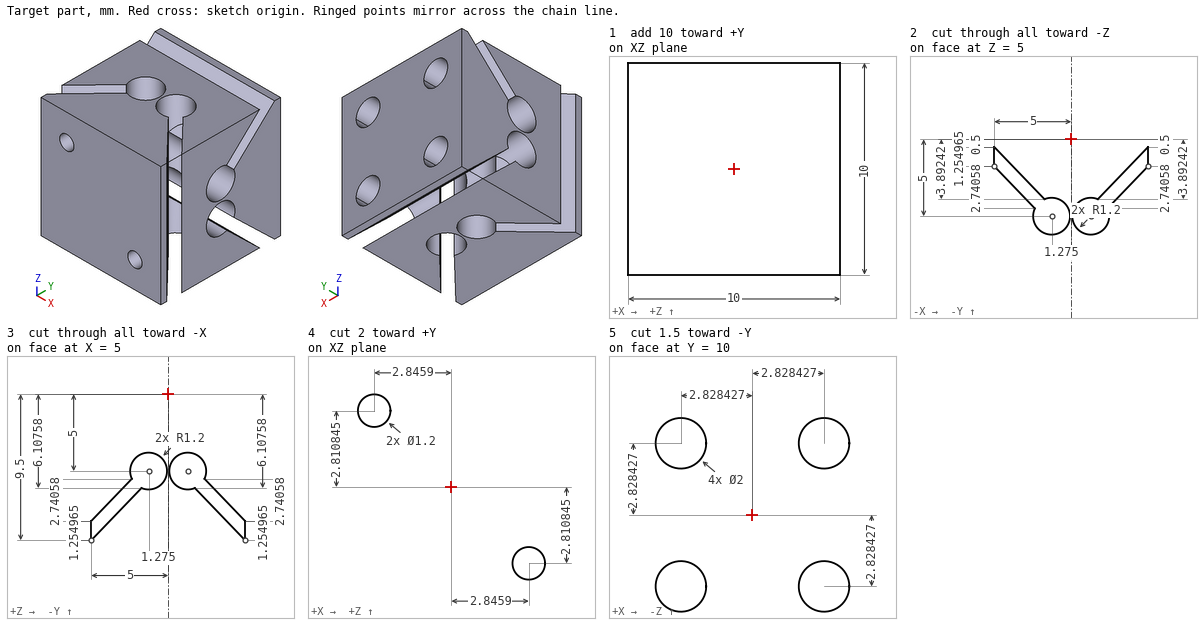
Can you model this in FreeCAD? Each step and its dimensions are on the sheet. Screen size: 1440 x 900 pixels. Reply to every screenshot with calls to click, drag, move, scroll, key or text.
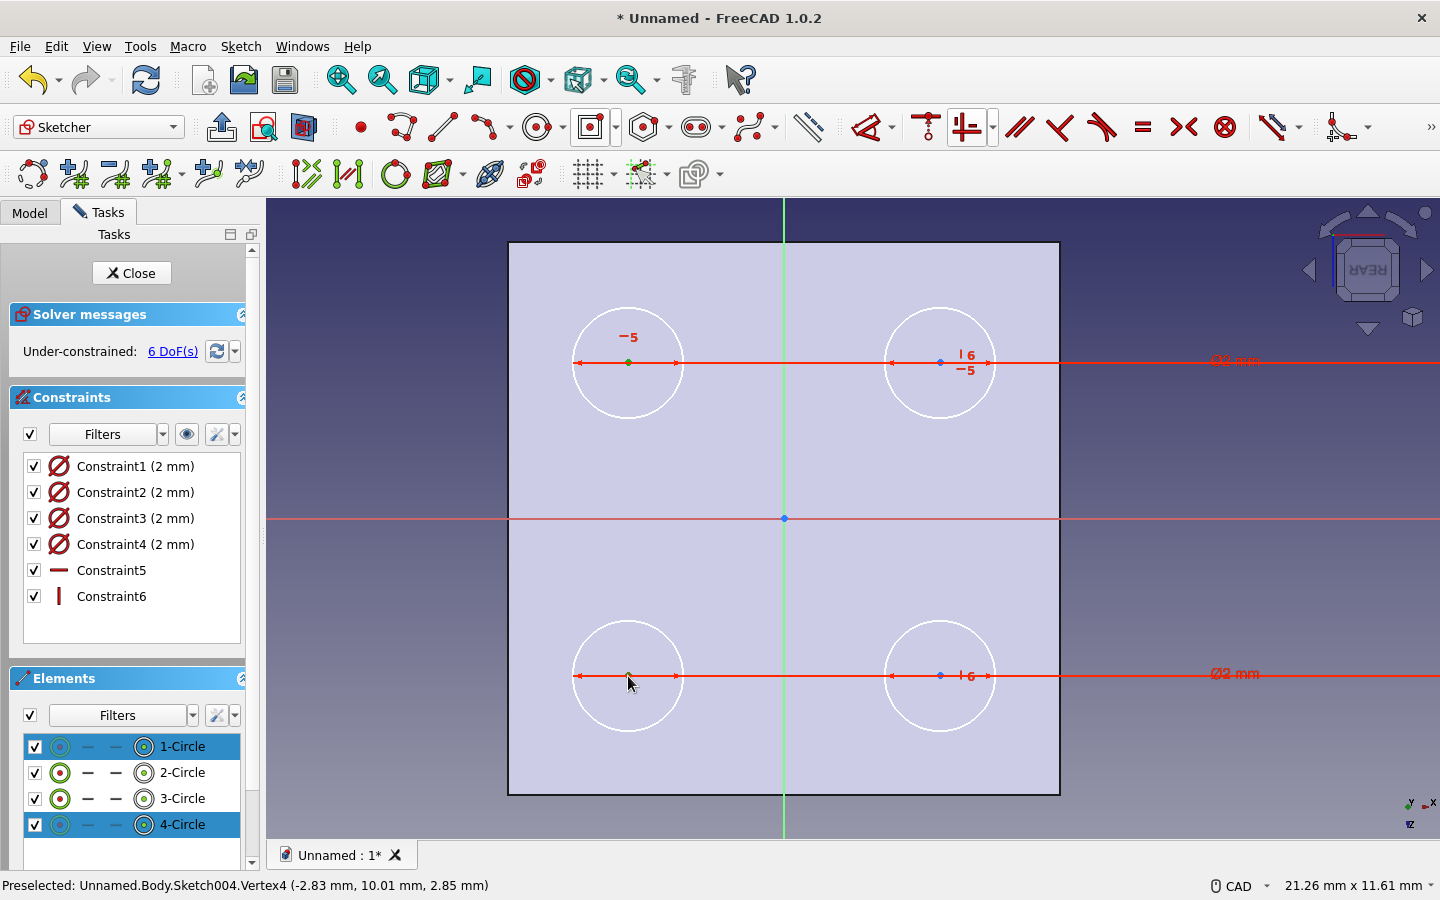
key(v)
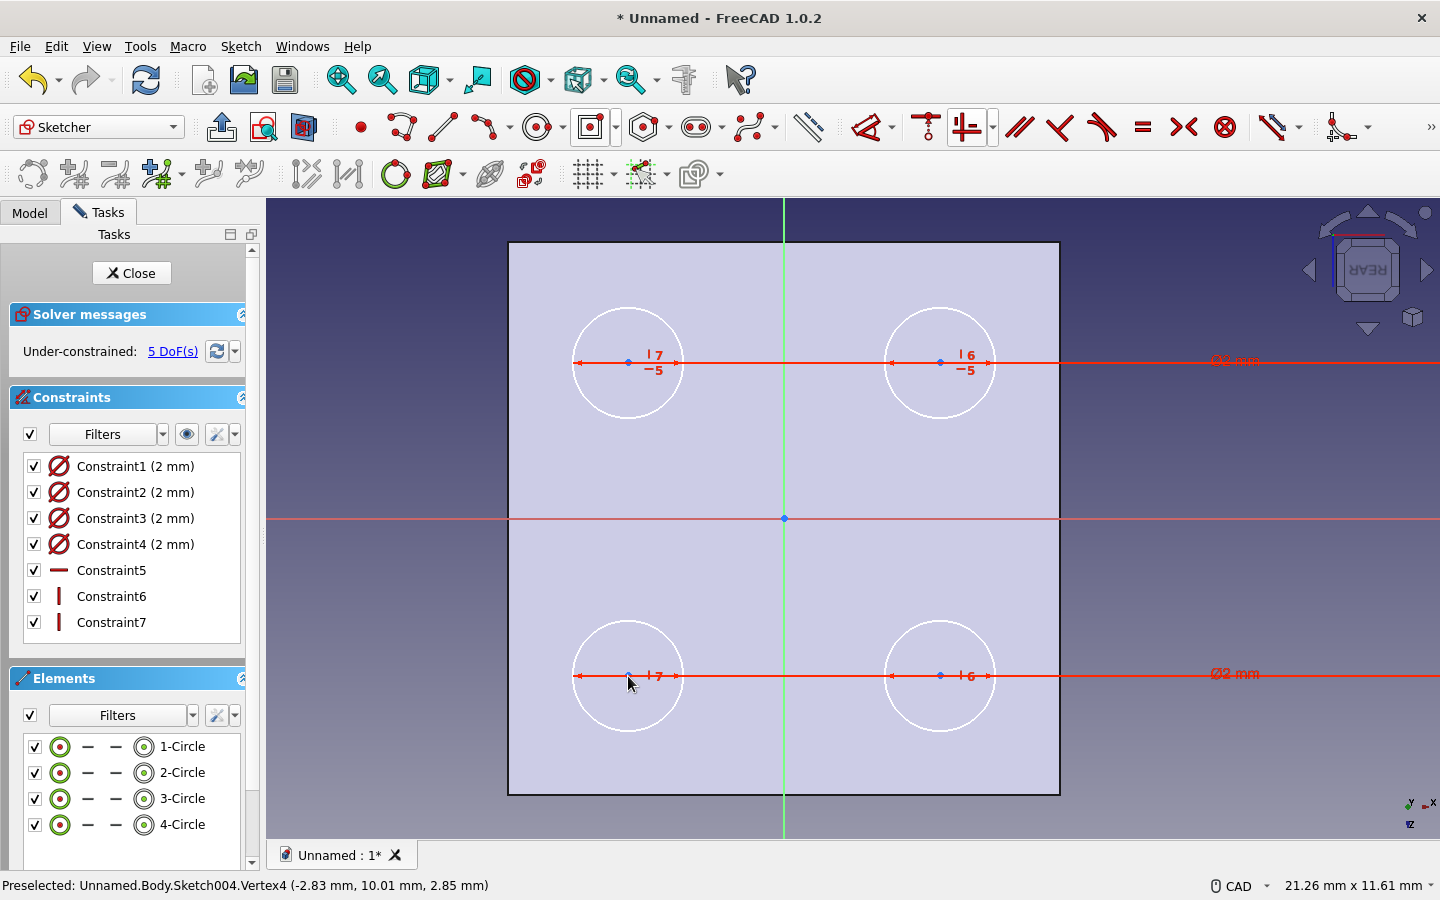
click(940, 676)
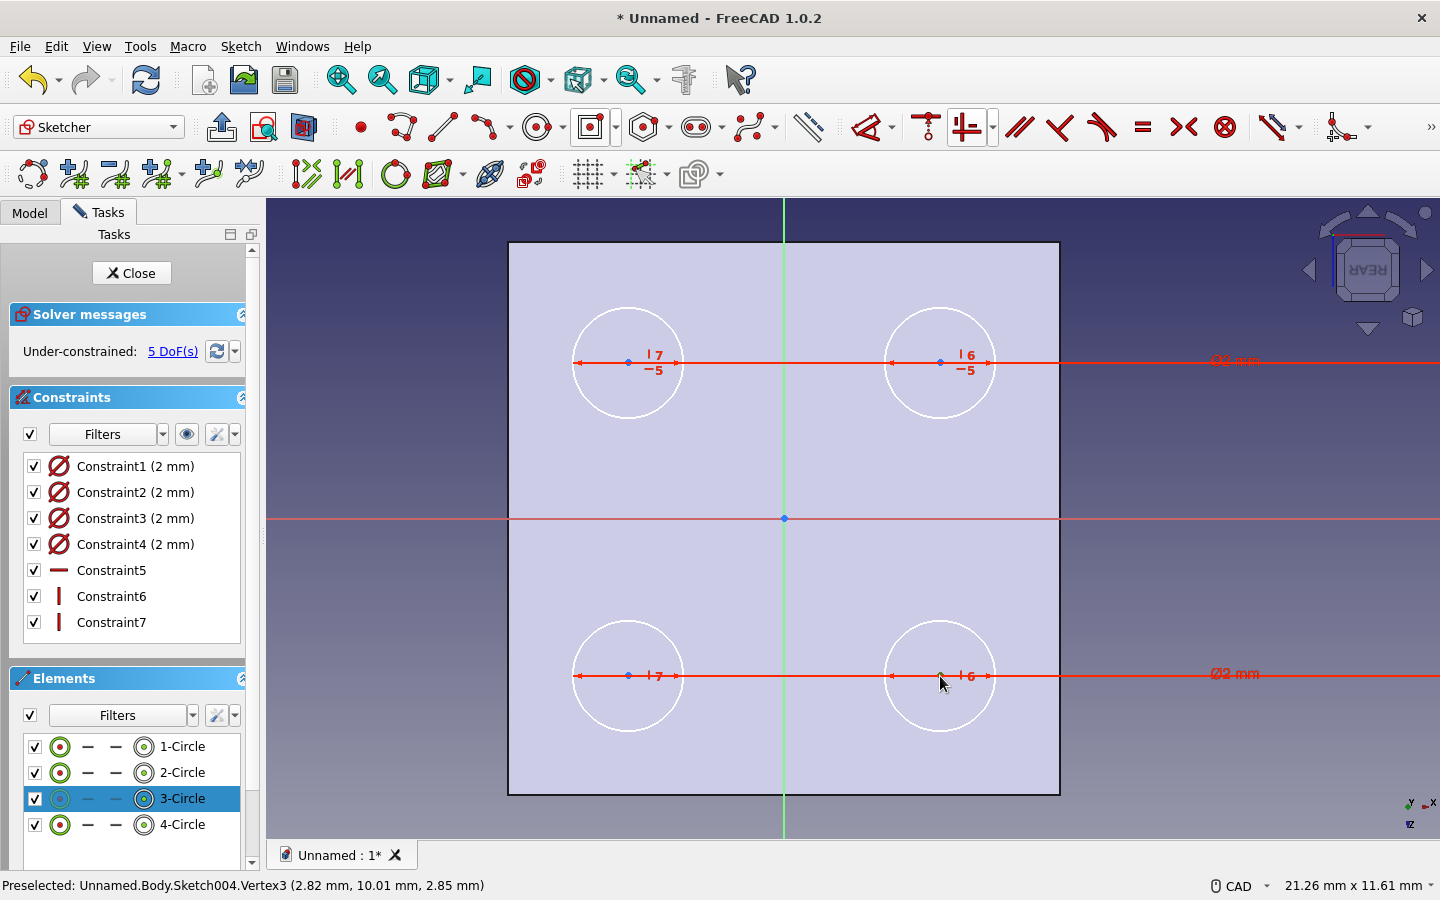
click(628, 676)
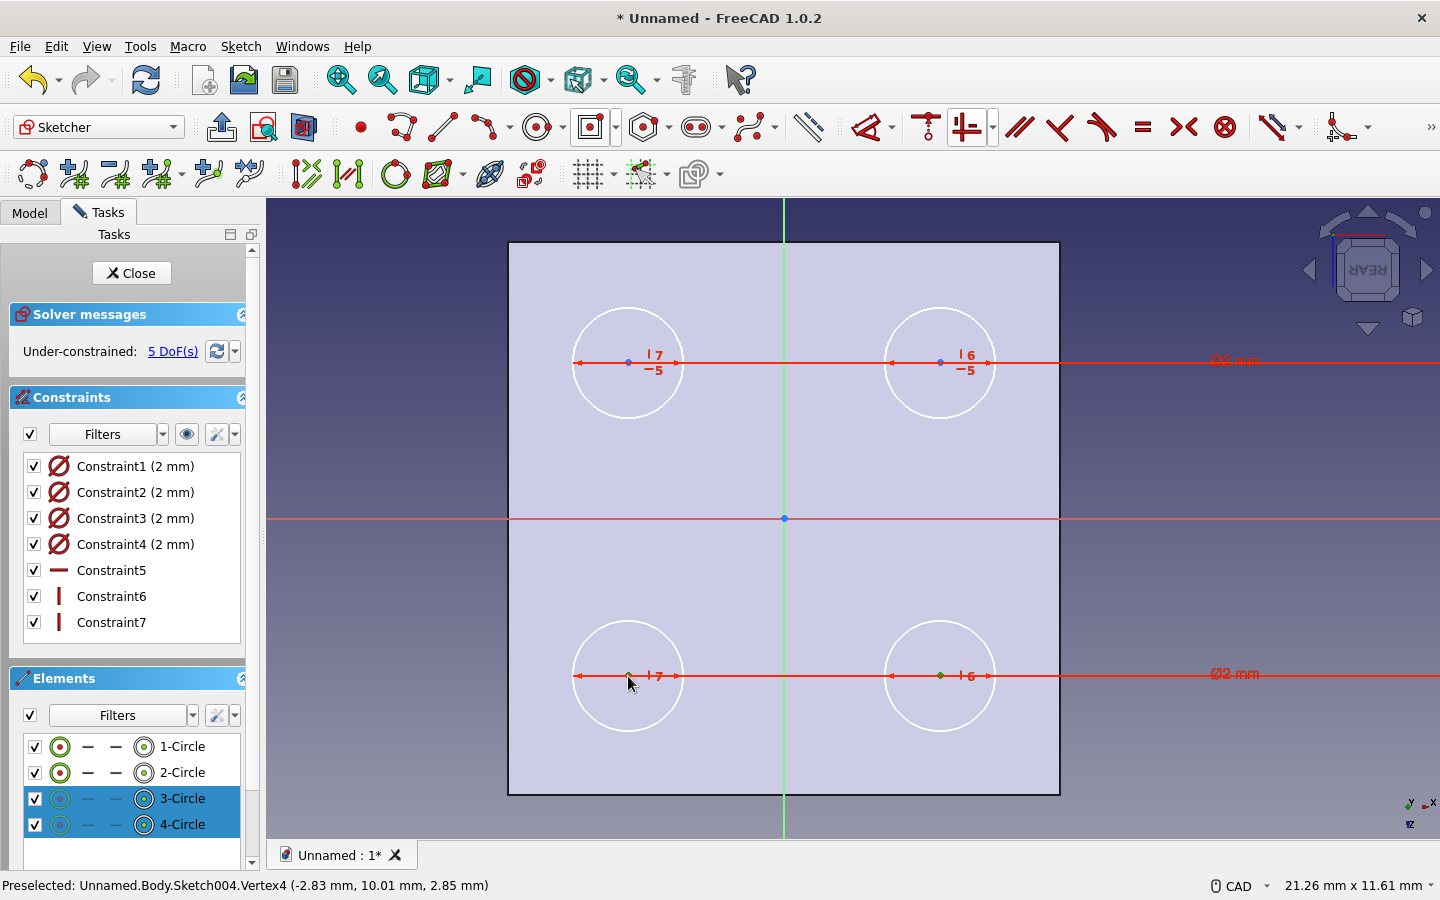
click(992, 128)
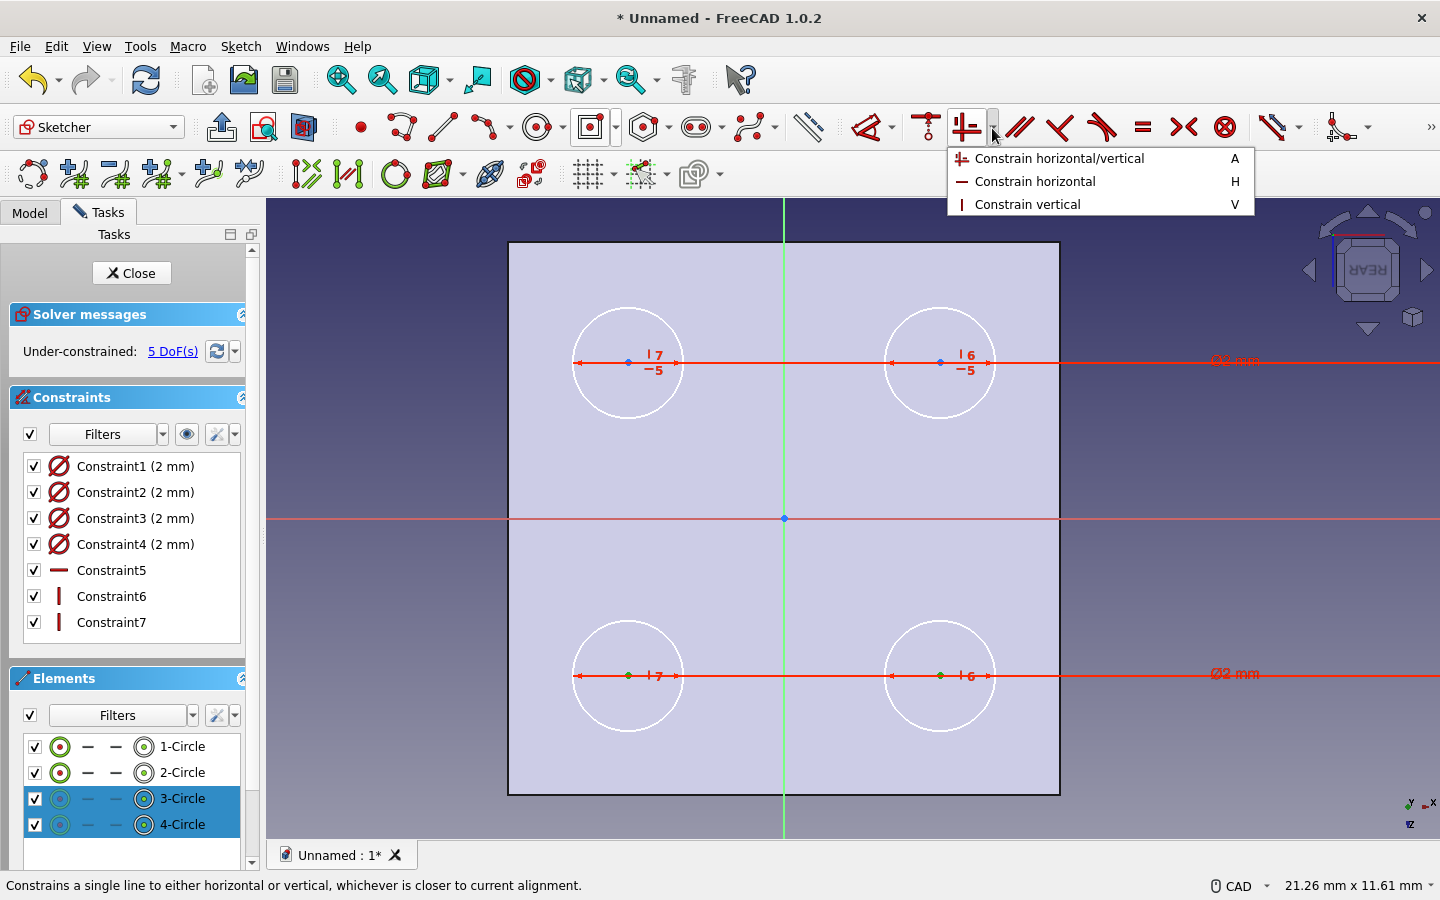
click(1101, 182)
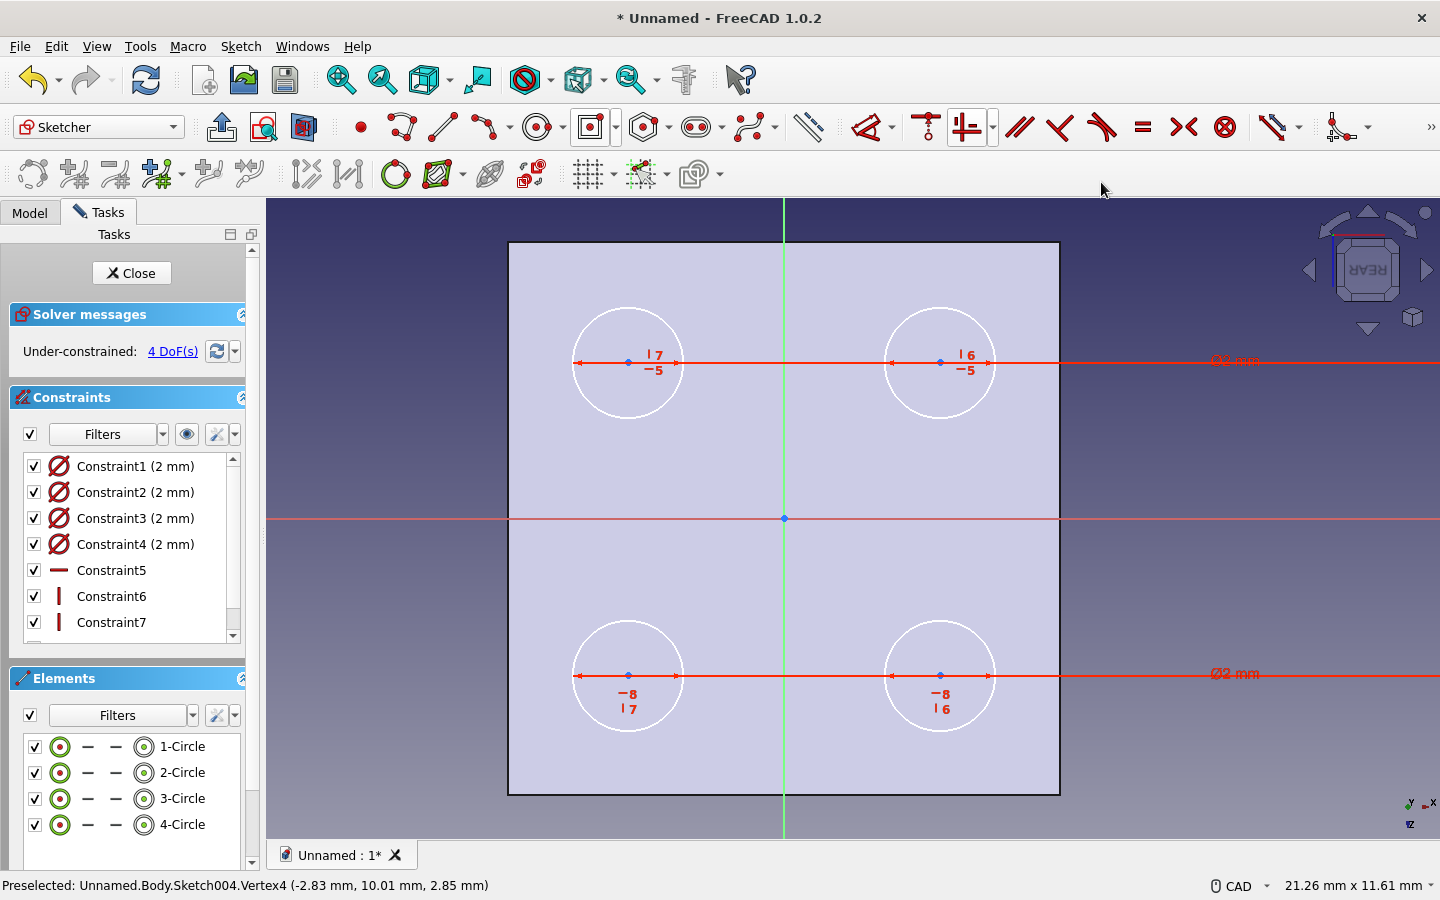
click(866, 128)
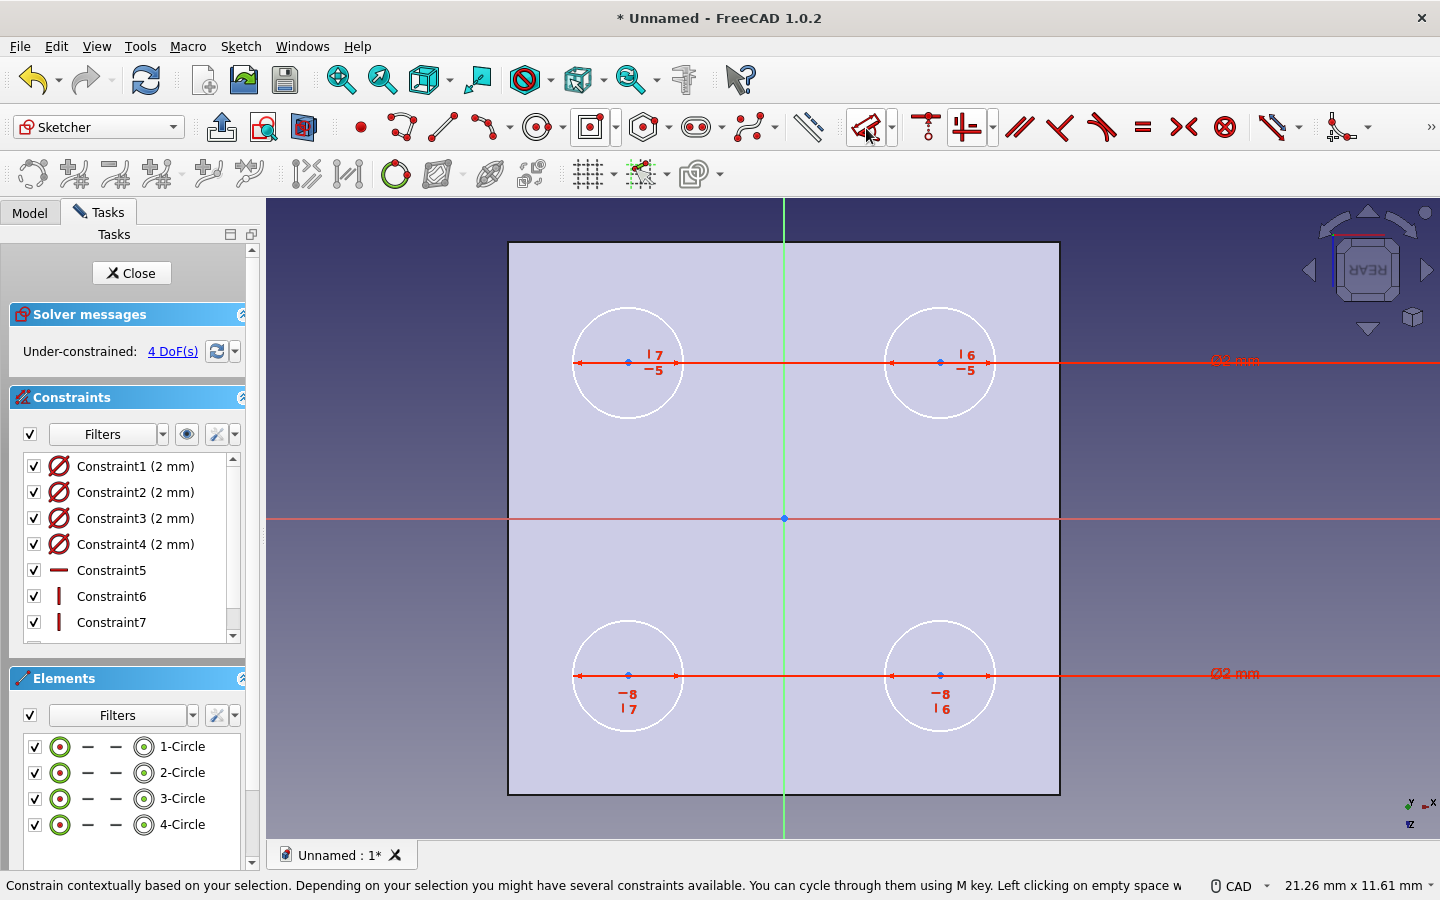
click(628, 363)
click(706, 329)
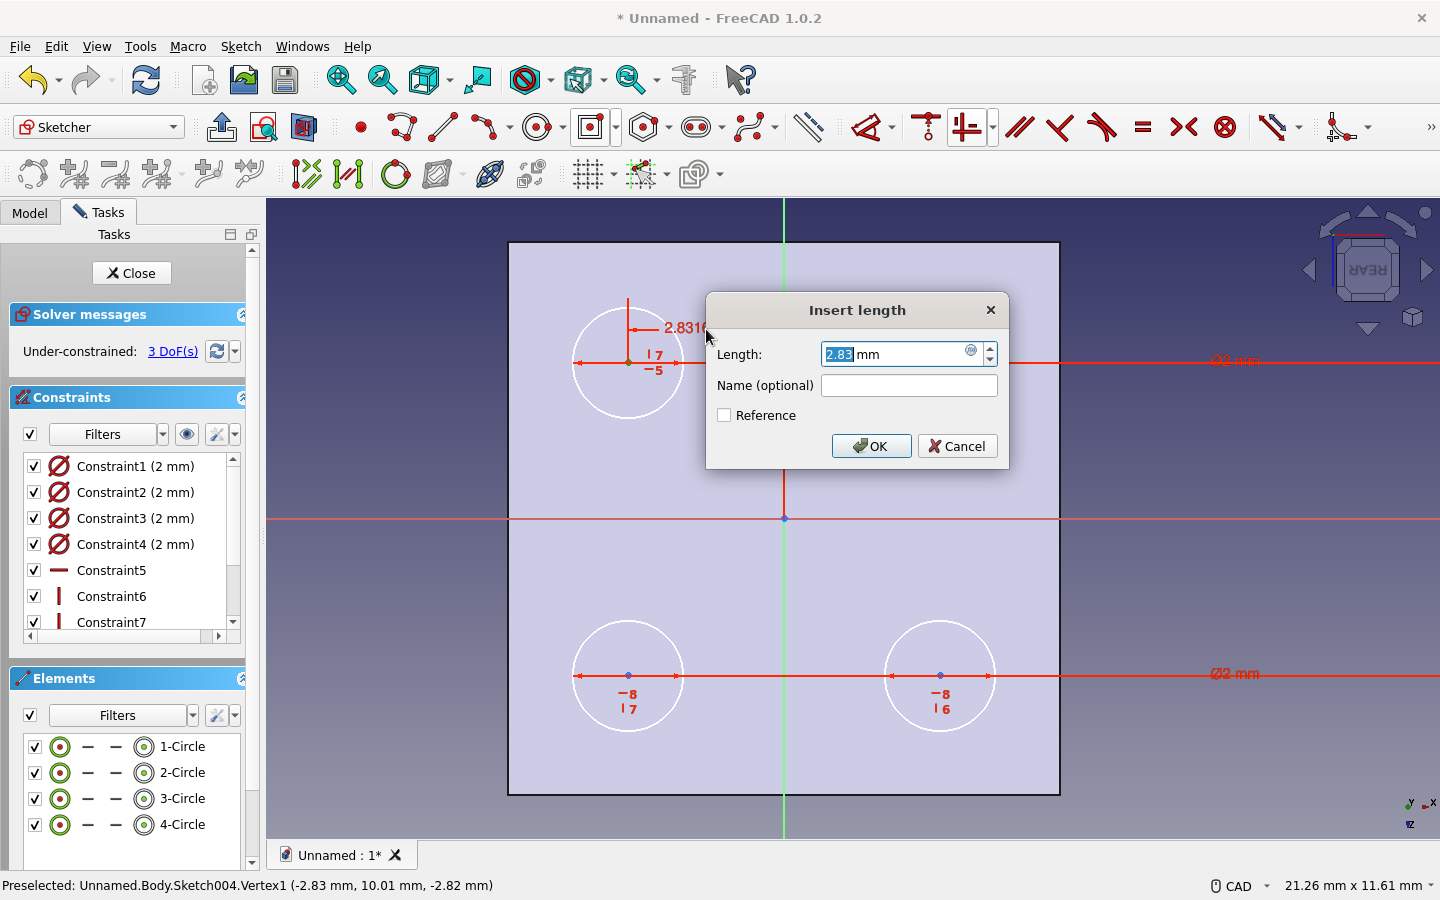
text(2.828427)
key(Return)